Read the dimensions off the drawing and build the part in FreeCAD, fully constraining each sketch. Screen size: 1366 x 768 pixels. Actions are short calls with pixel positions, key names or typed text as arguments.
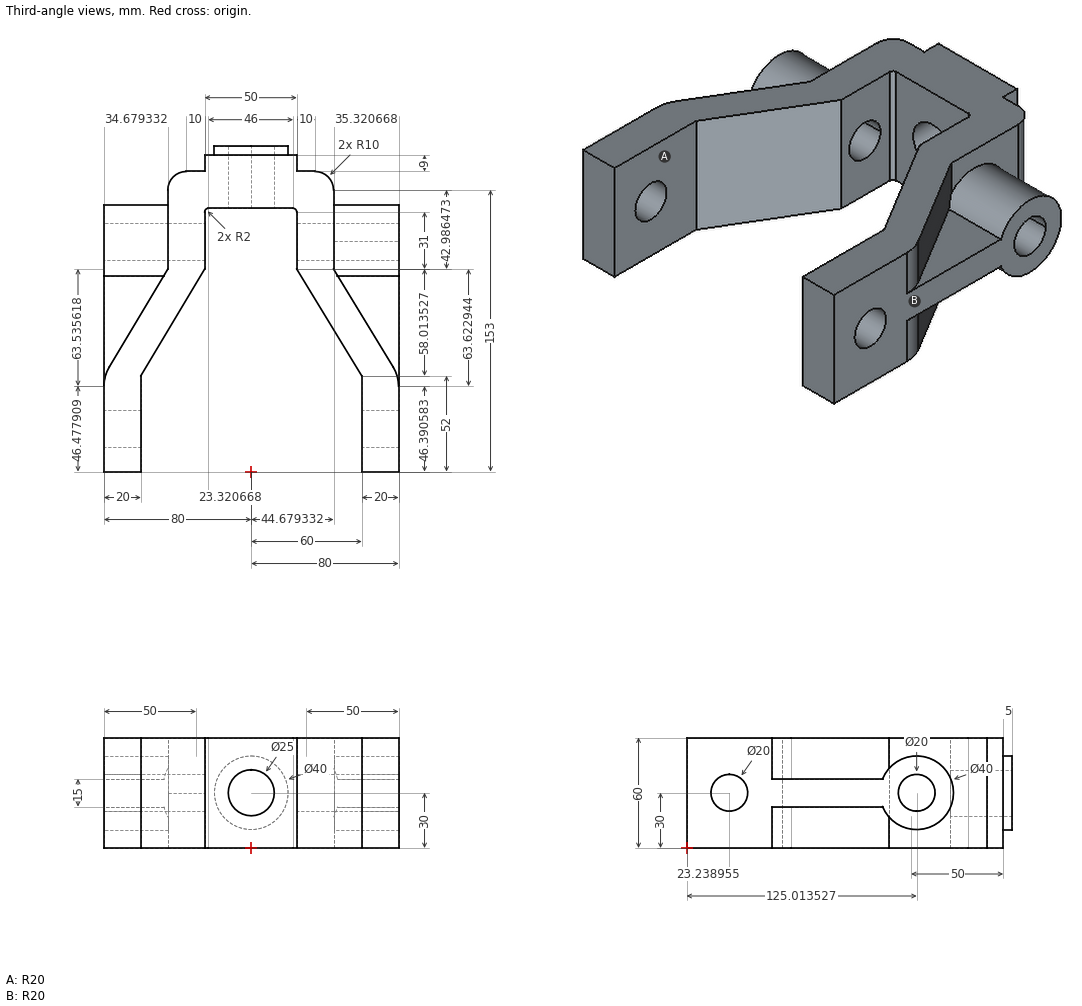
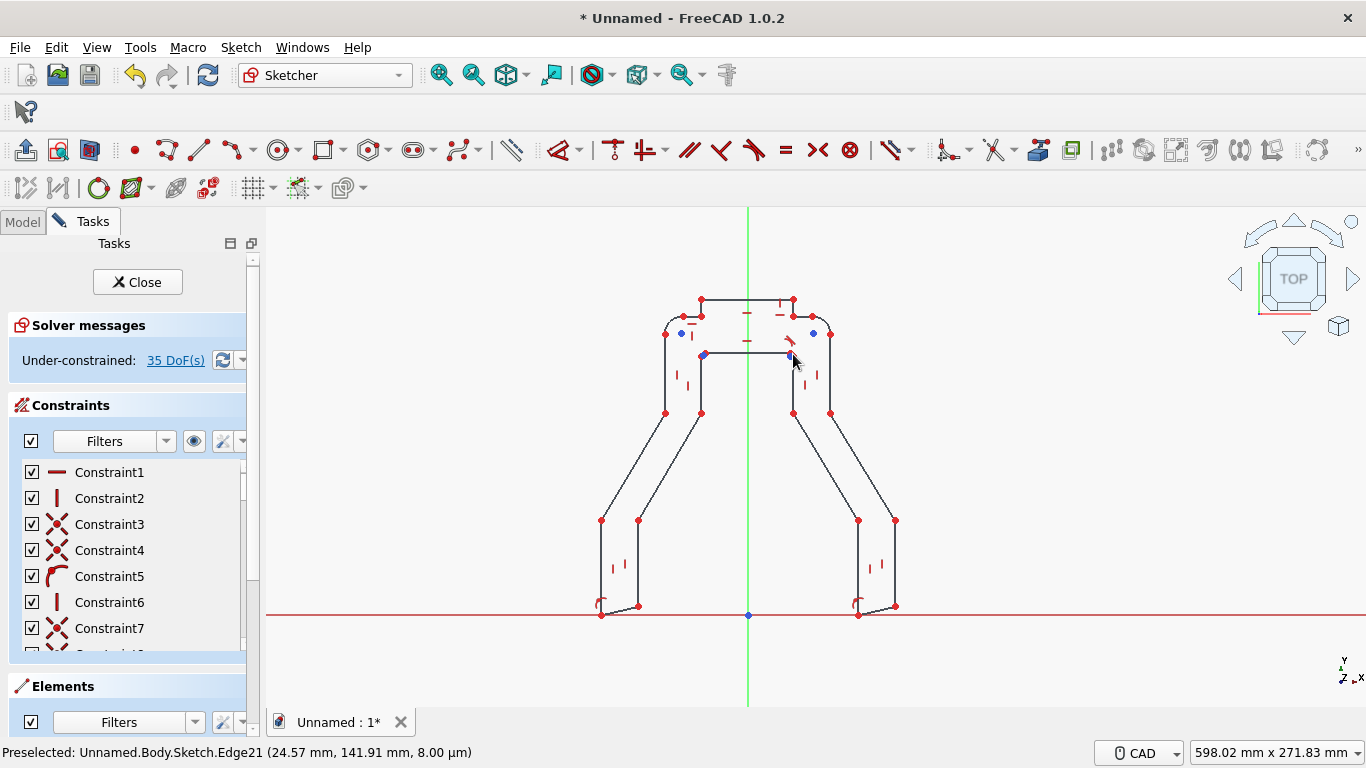
click(731, 353)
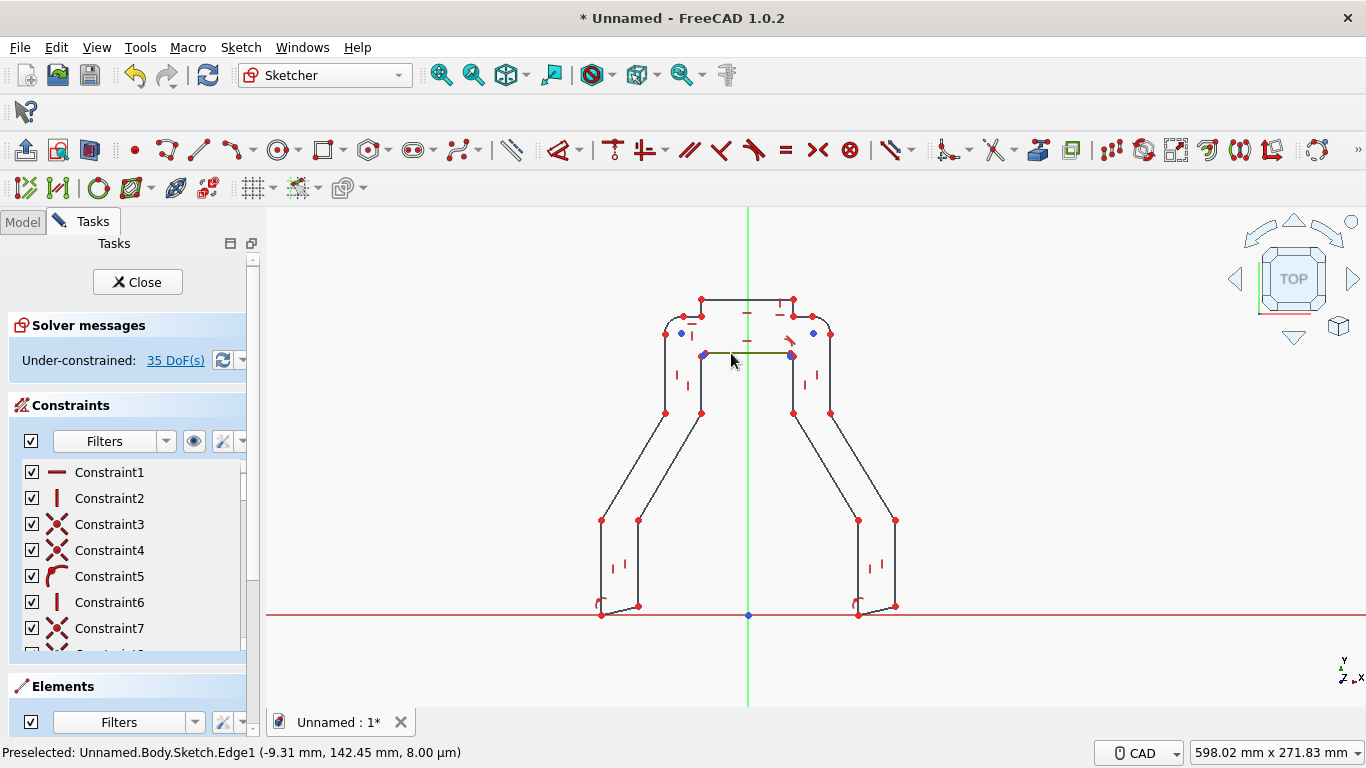
scroll(702, 354, up, 9)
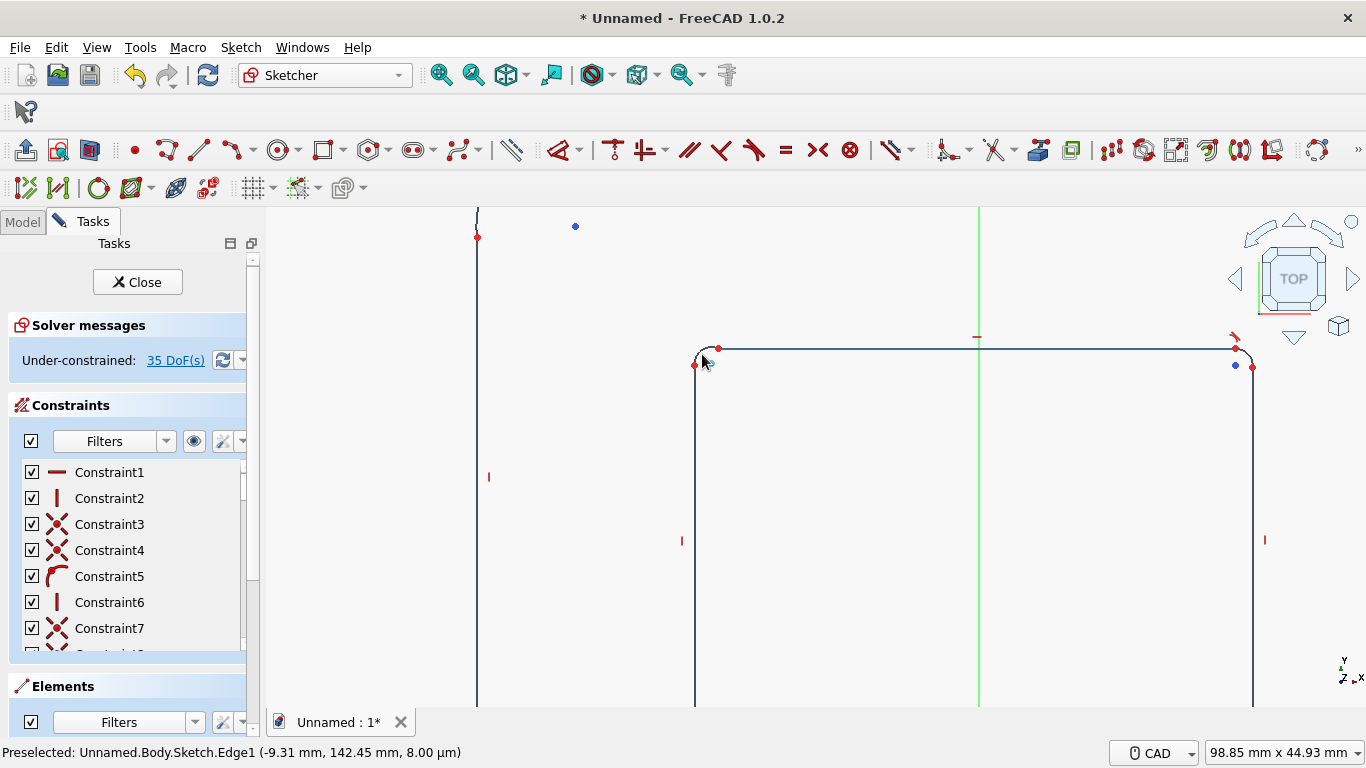
click(702, 350)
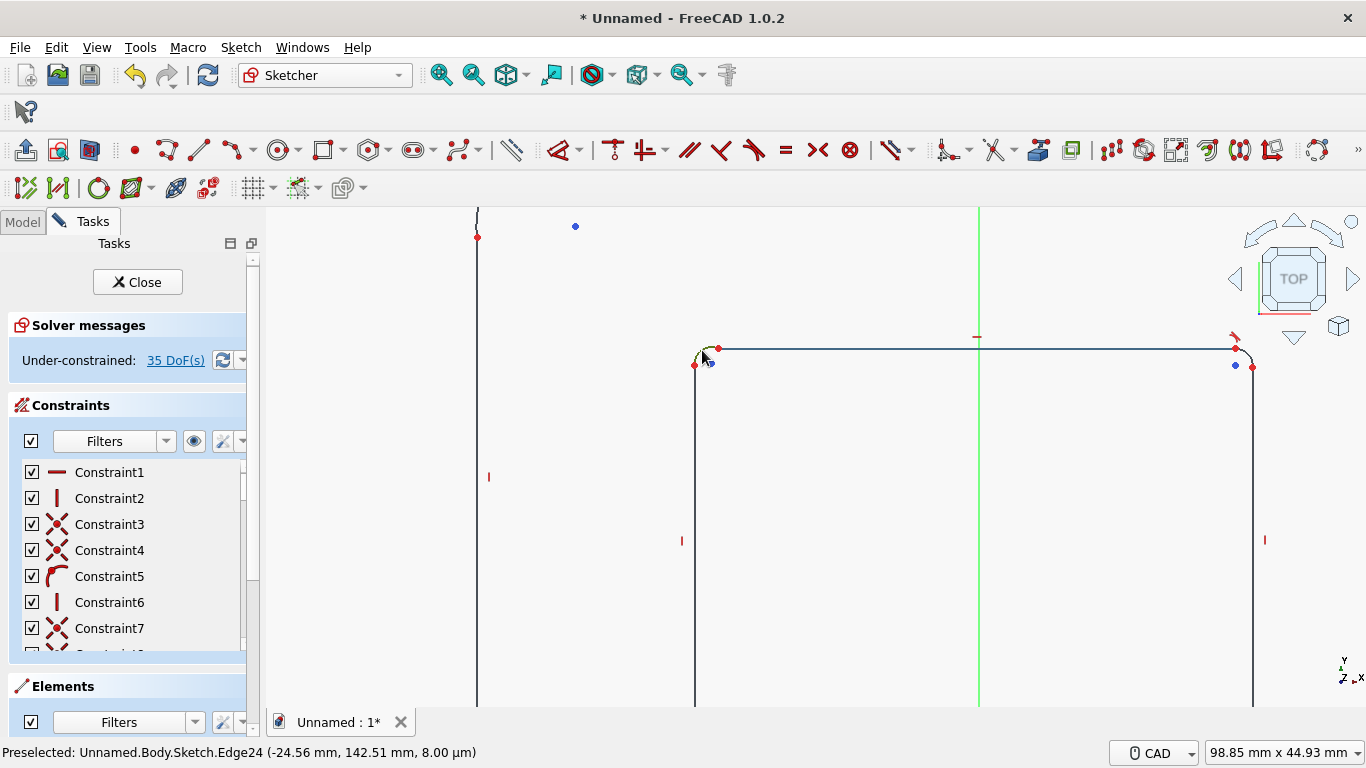
key(t)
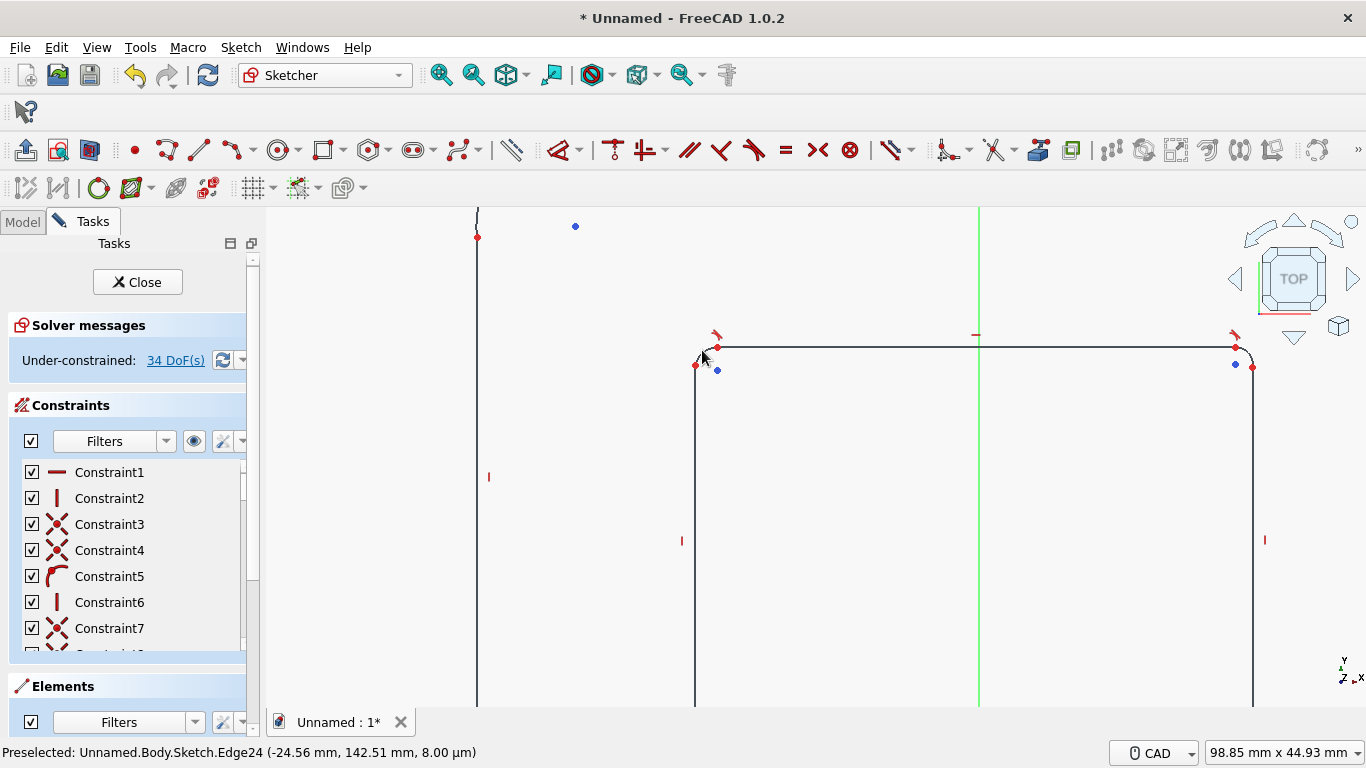
scroll(702, 354, down, 9)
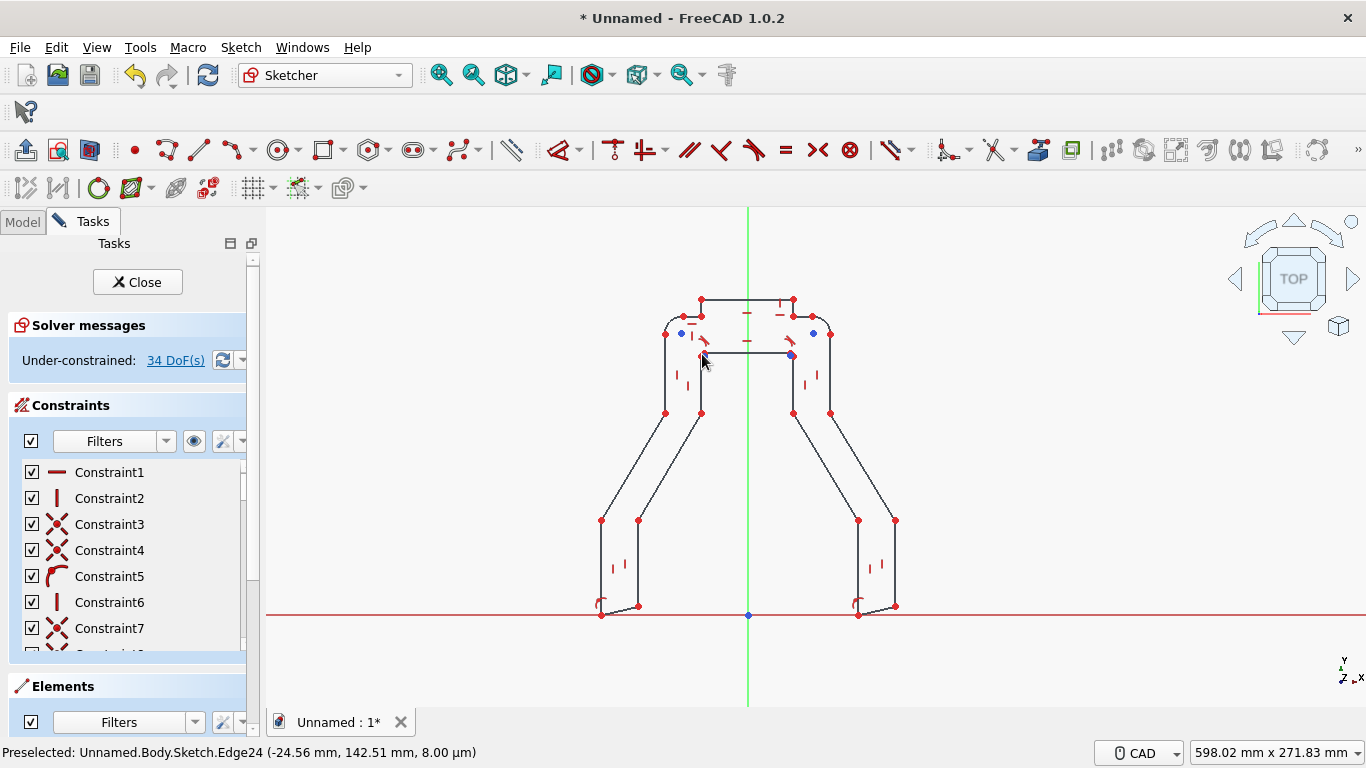
click(793, 373)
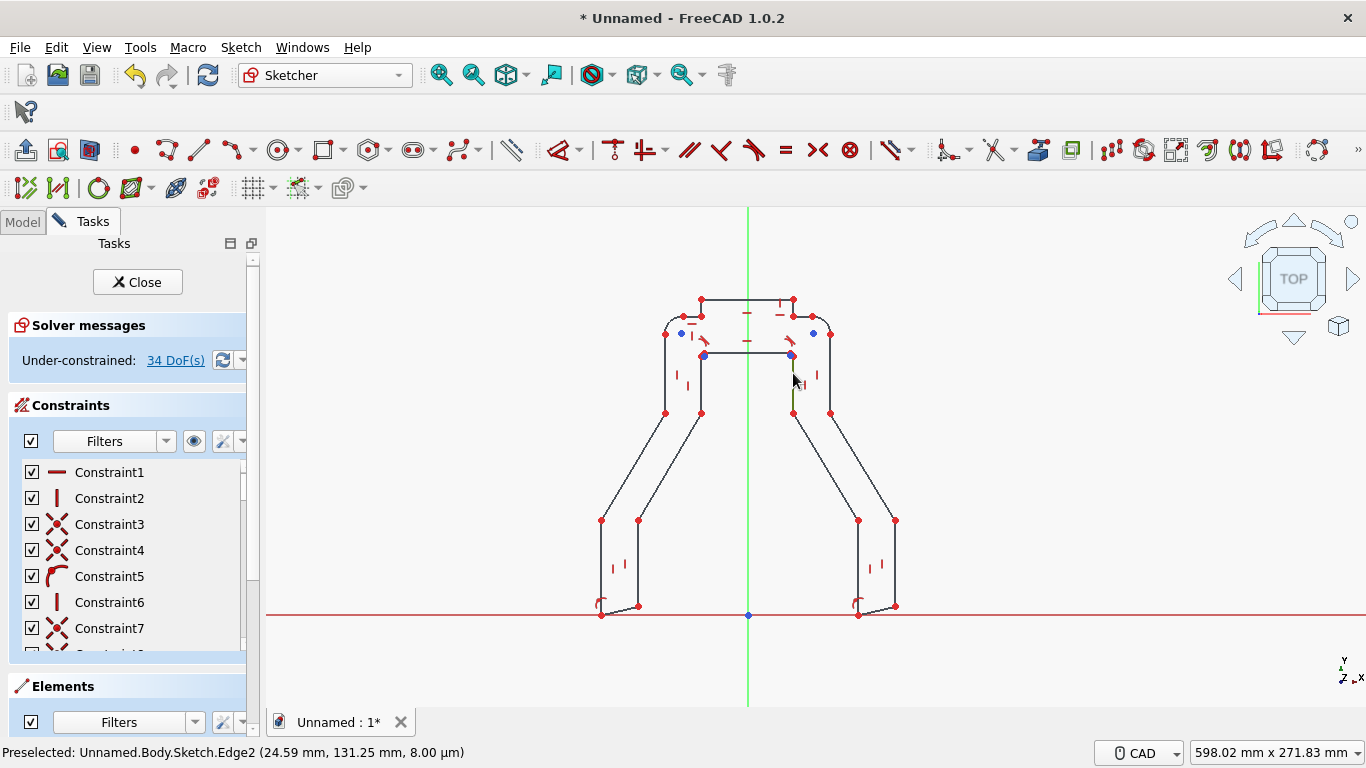
scroll(793, 354, up, 9)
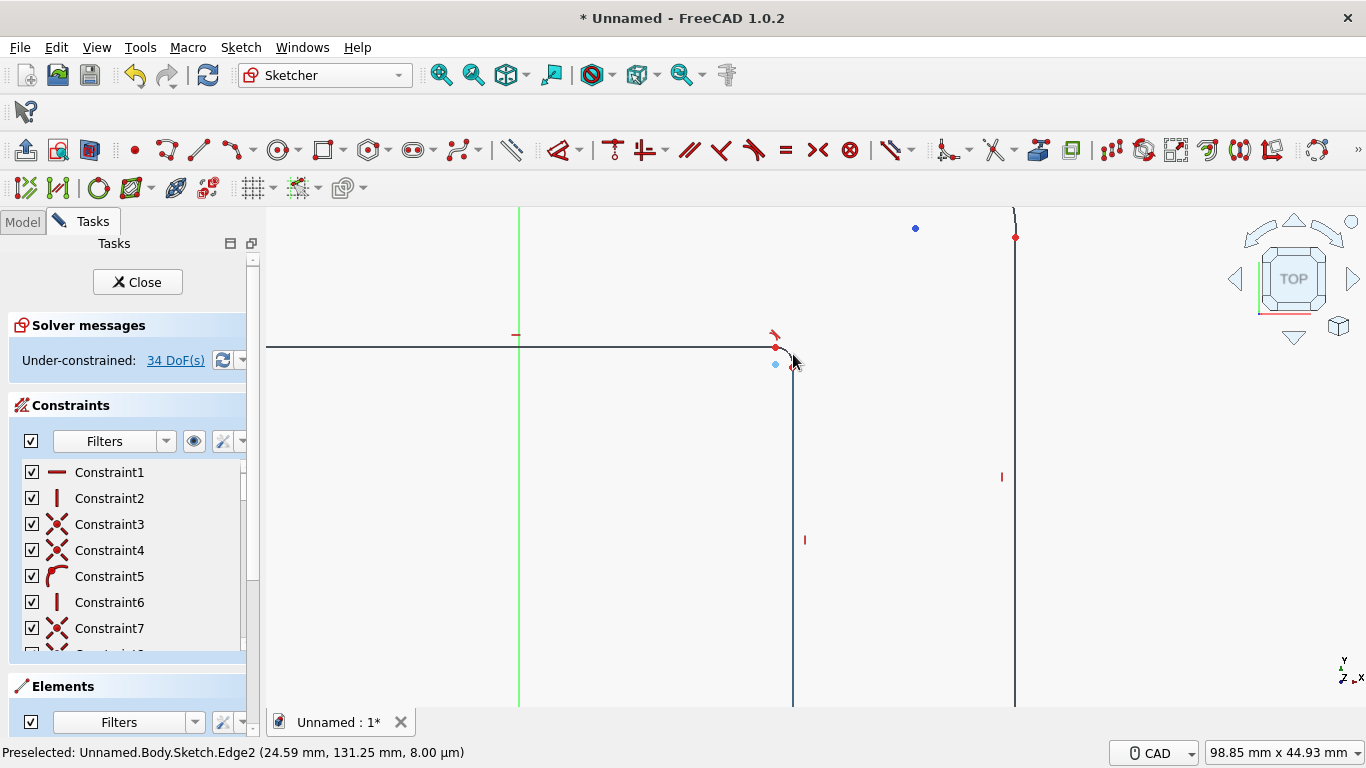
click(789, 353)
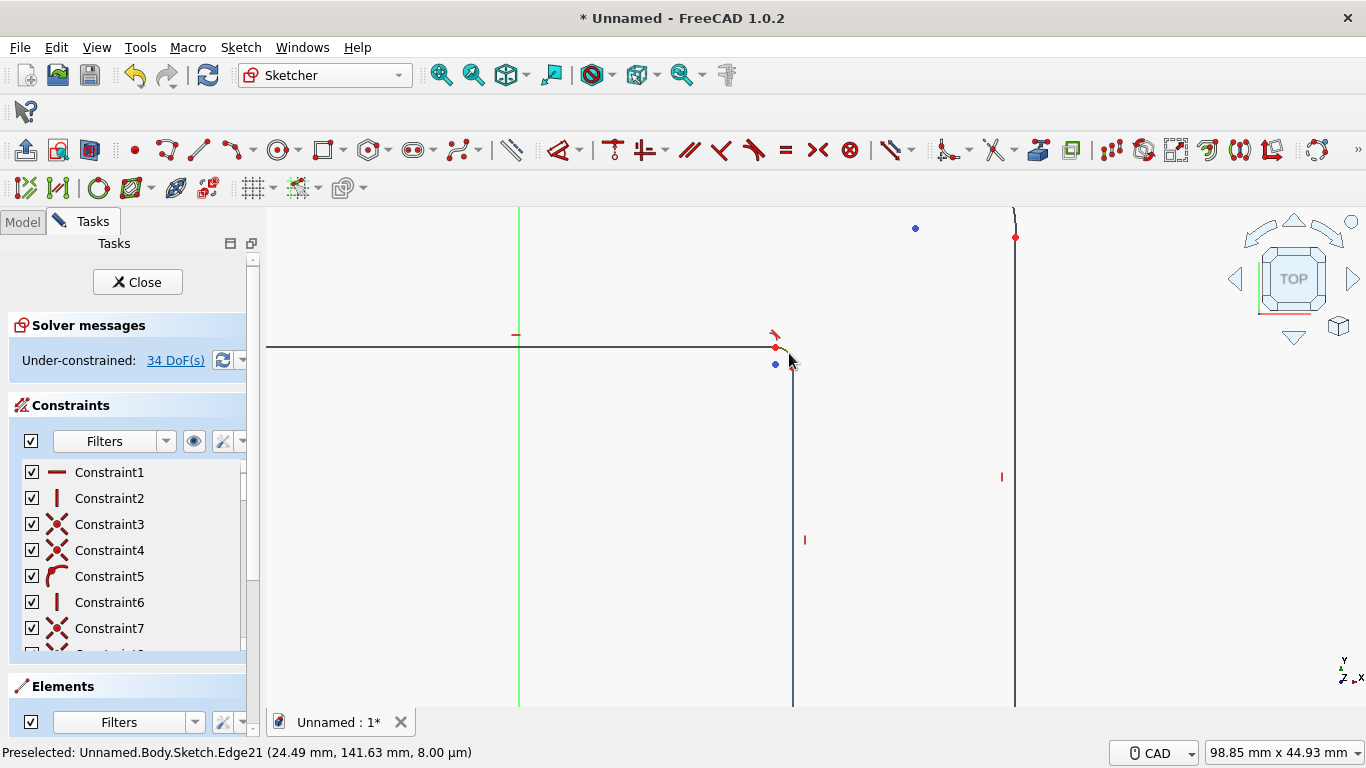
key(t)